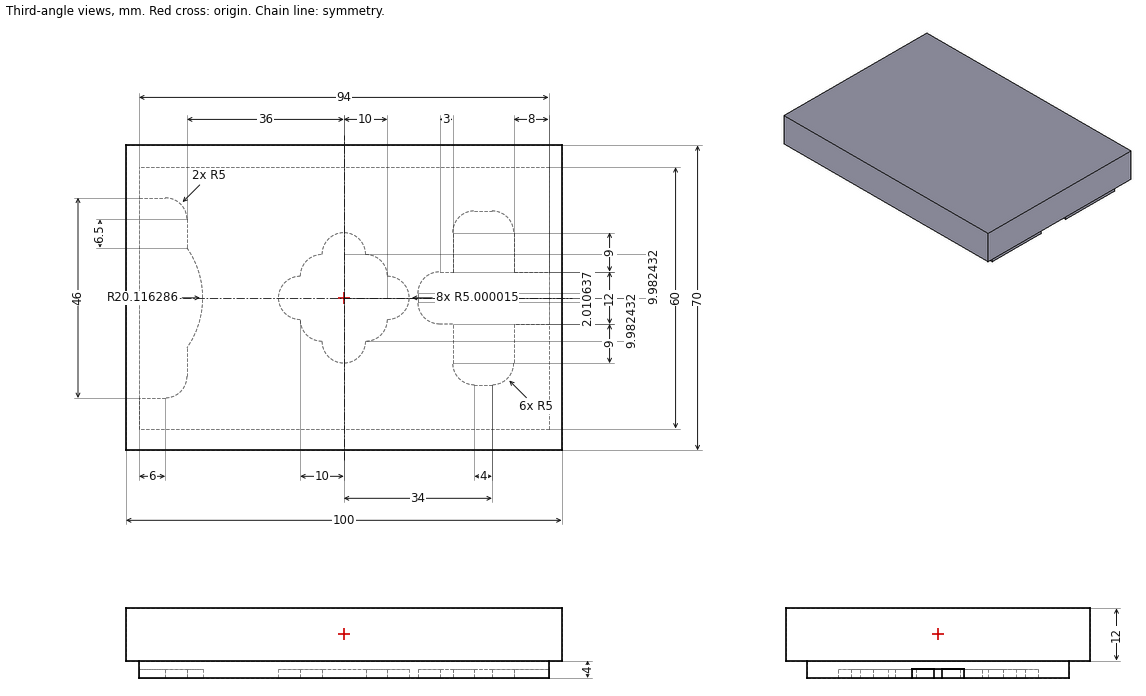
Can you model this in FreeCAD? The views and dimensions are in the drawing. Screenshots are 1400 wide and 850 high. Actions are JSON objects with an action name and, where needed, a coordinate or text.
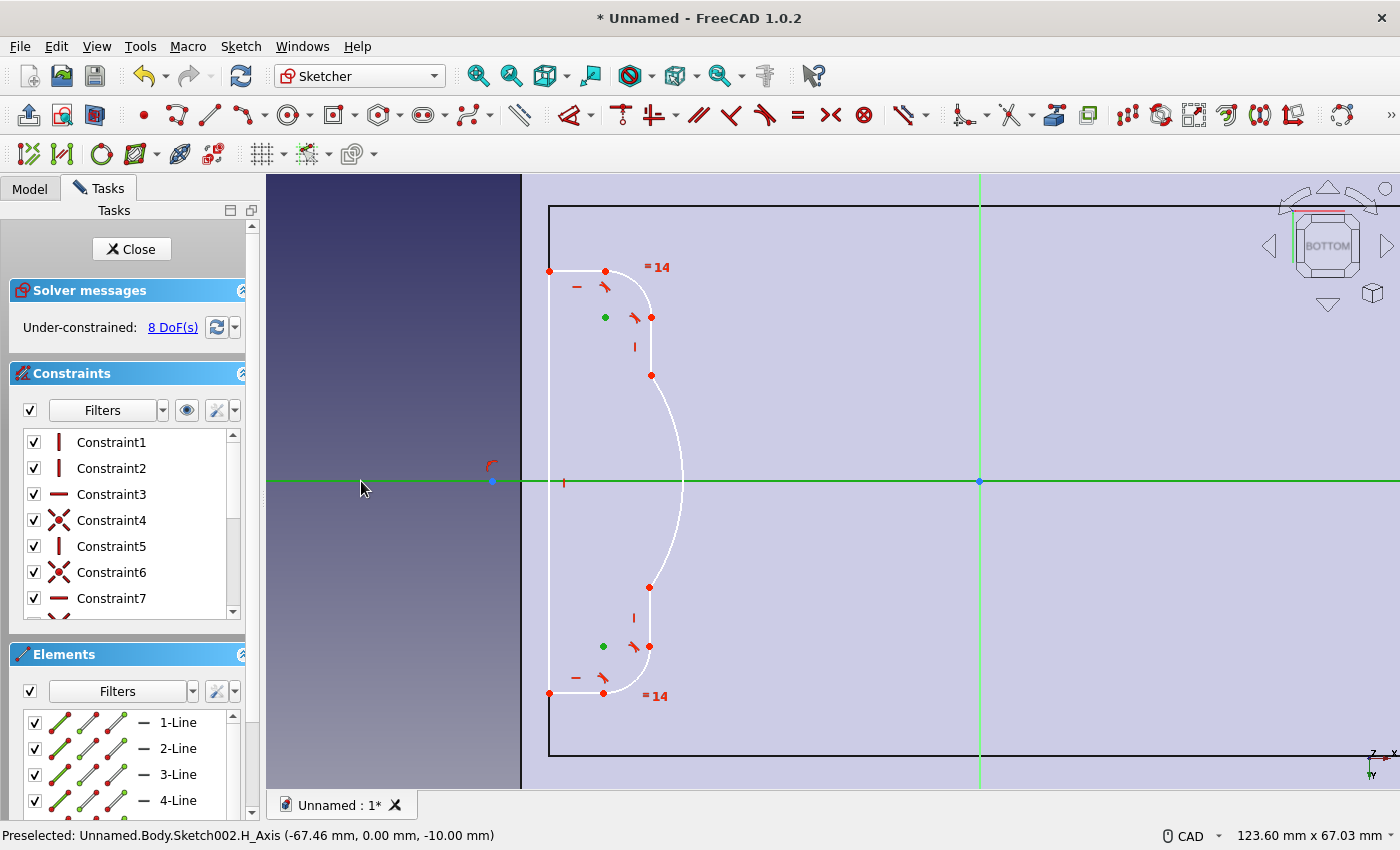
{"action": "left_click", "coordinate": [831, 116]}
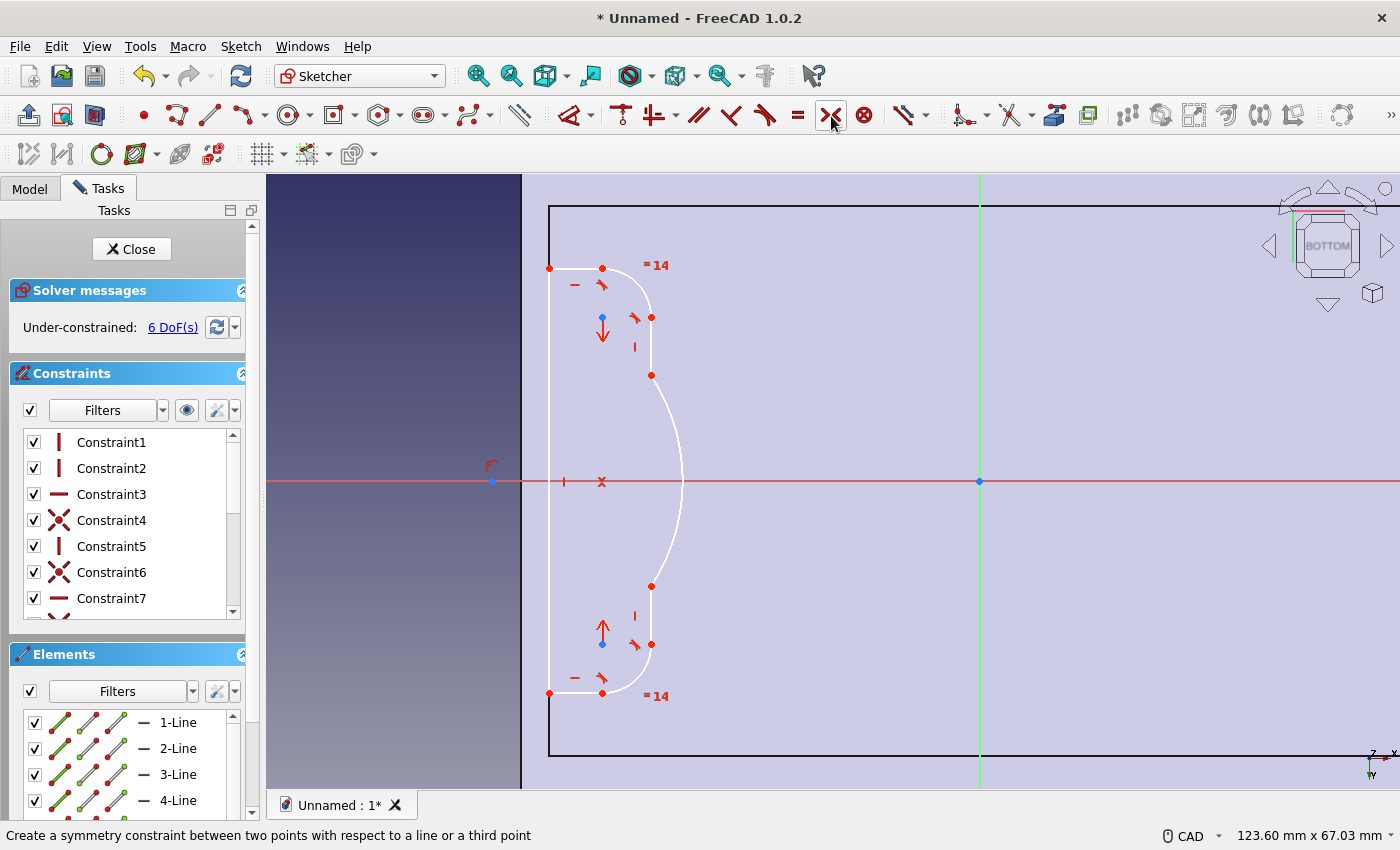
{"action": "left_click", "coordinate": [568, 116]}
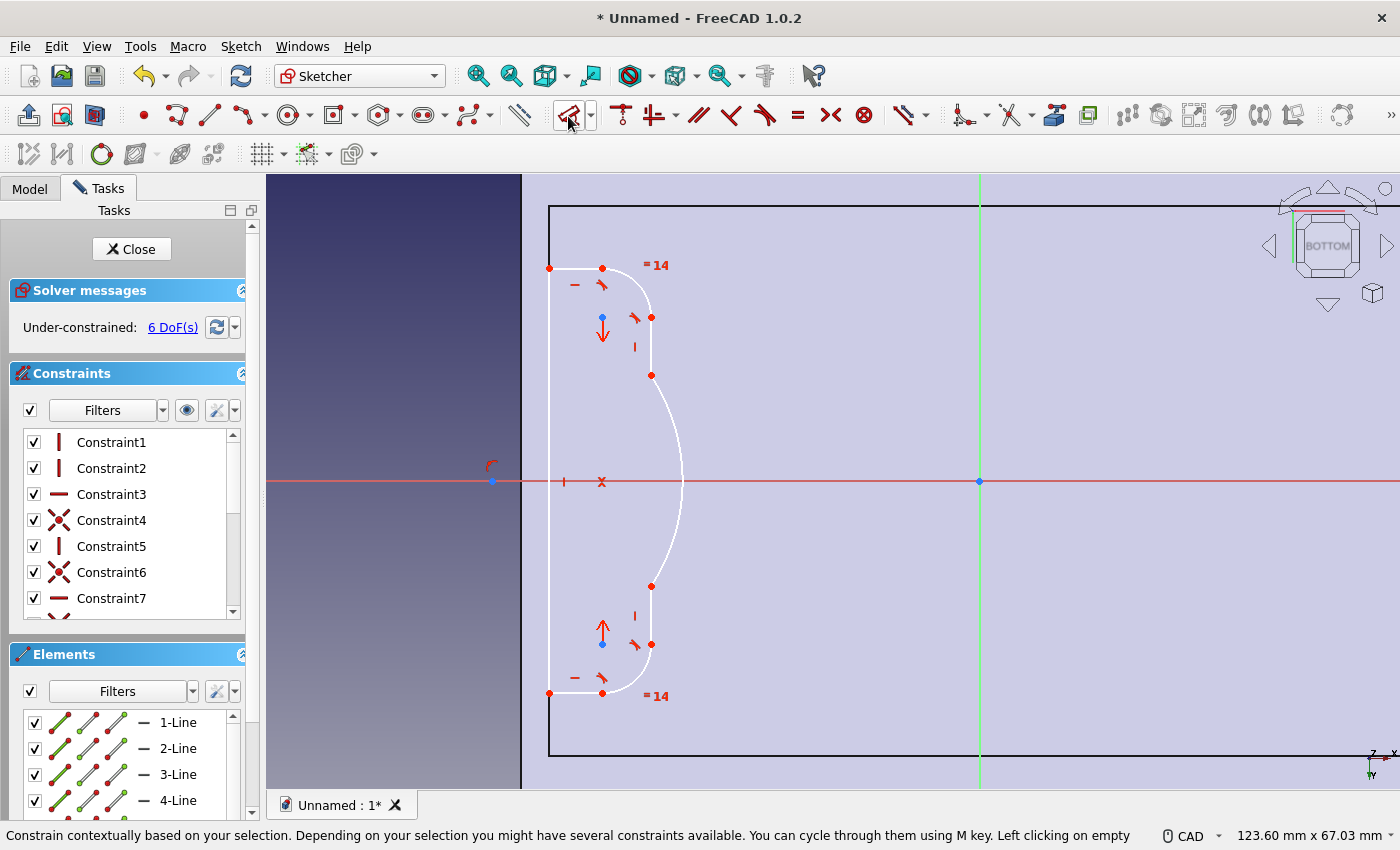
{"action": "left_click", "coordinate": [677, 525]}
{"action": "left_click", "coordinate": [708, 532]}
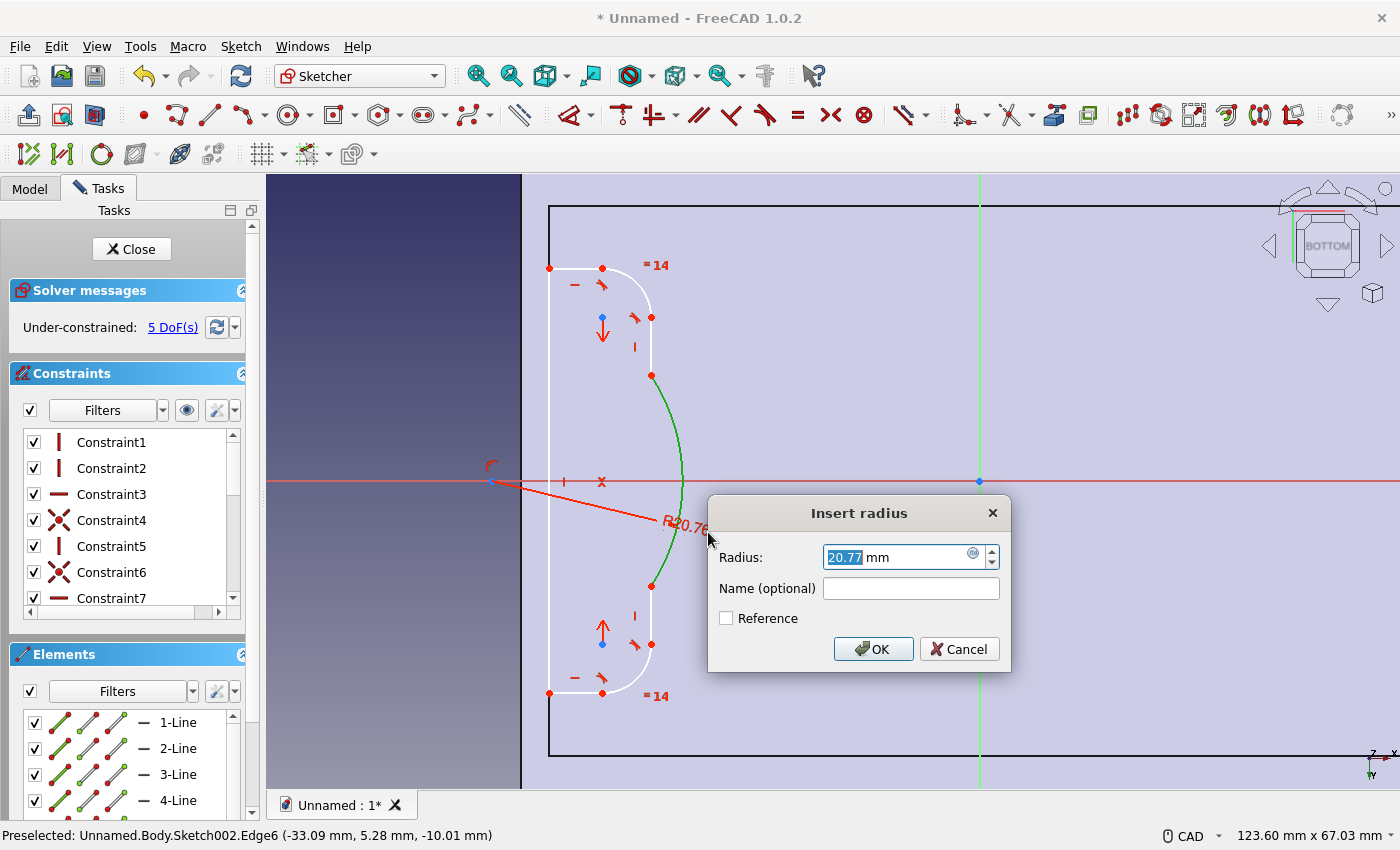
{"action": "type", "text": "20.116286"}
{"action": "key", "text": "Return"}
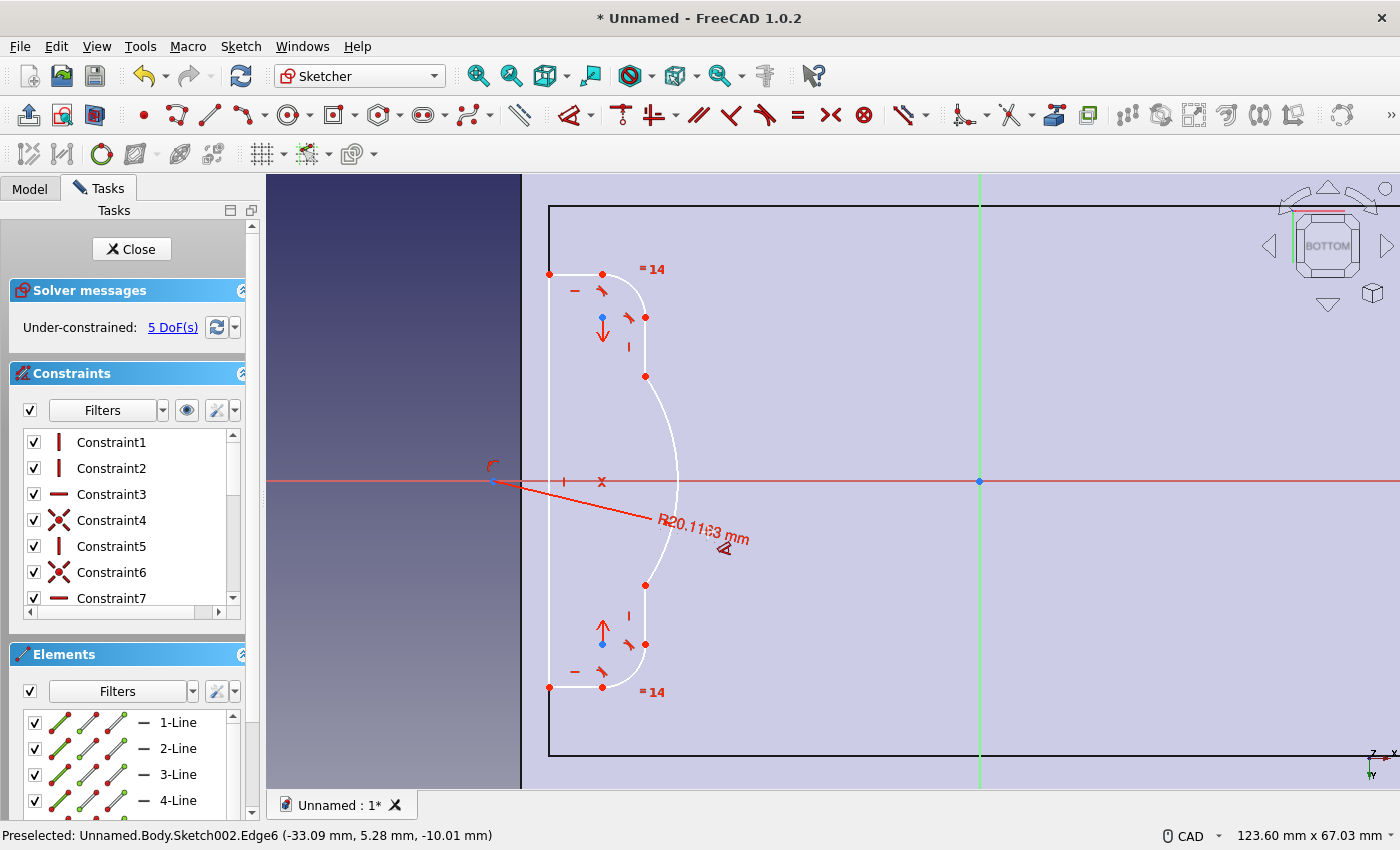
{"action": "left_click", "coordinate": [641, 298]}
{"action": "left_click", "coordinate": [670, 284]}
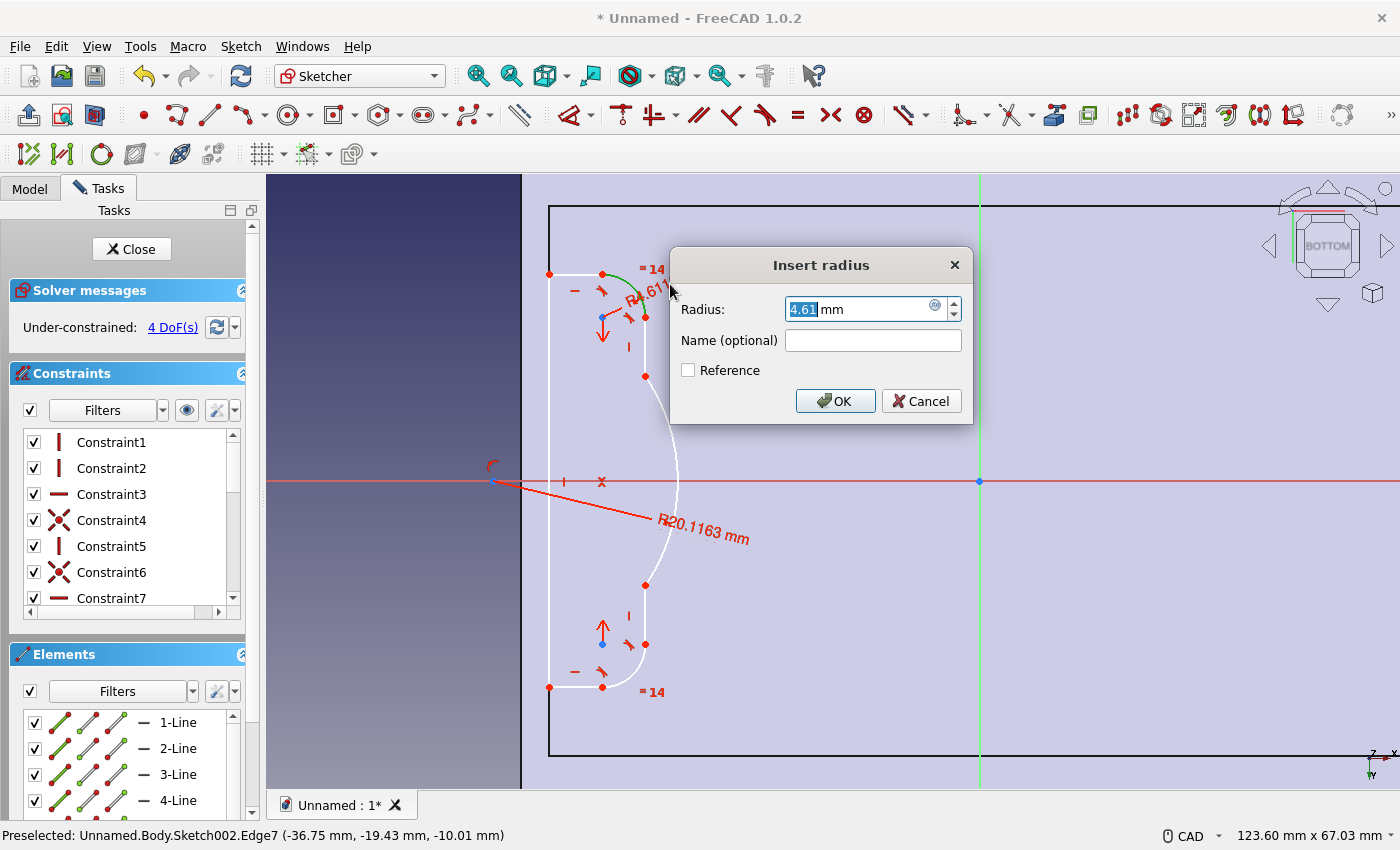
{"action": "type", "text": "5"}
{"action": "key", "text": "Return"}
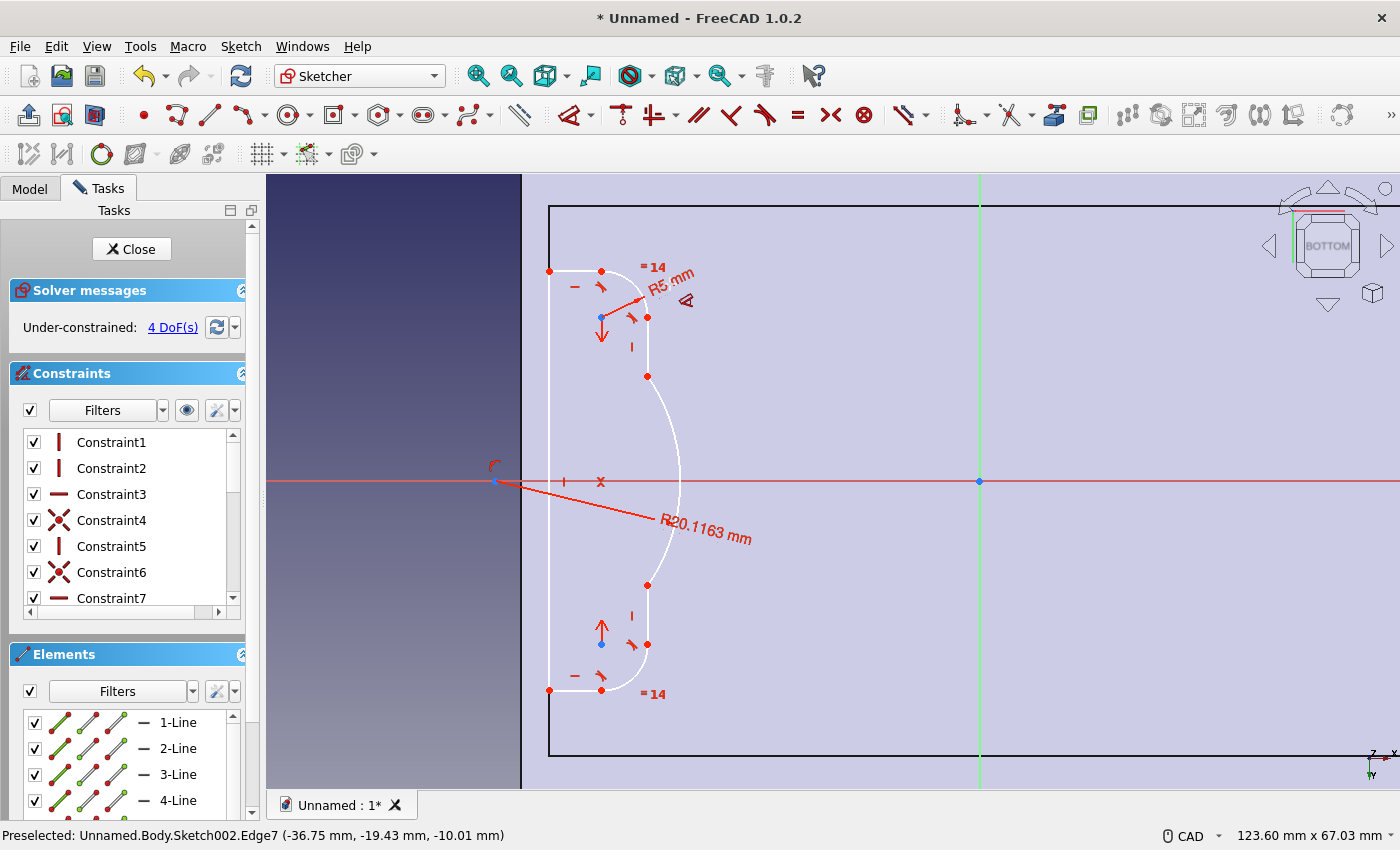
{"action": "left_click", "coordinate": [586, 271]}
{"action": "left_click", "coordinate": [575, 237]}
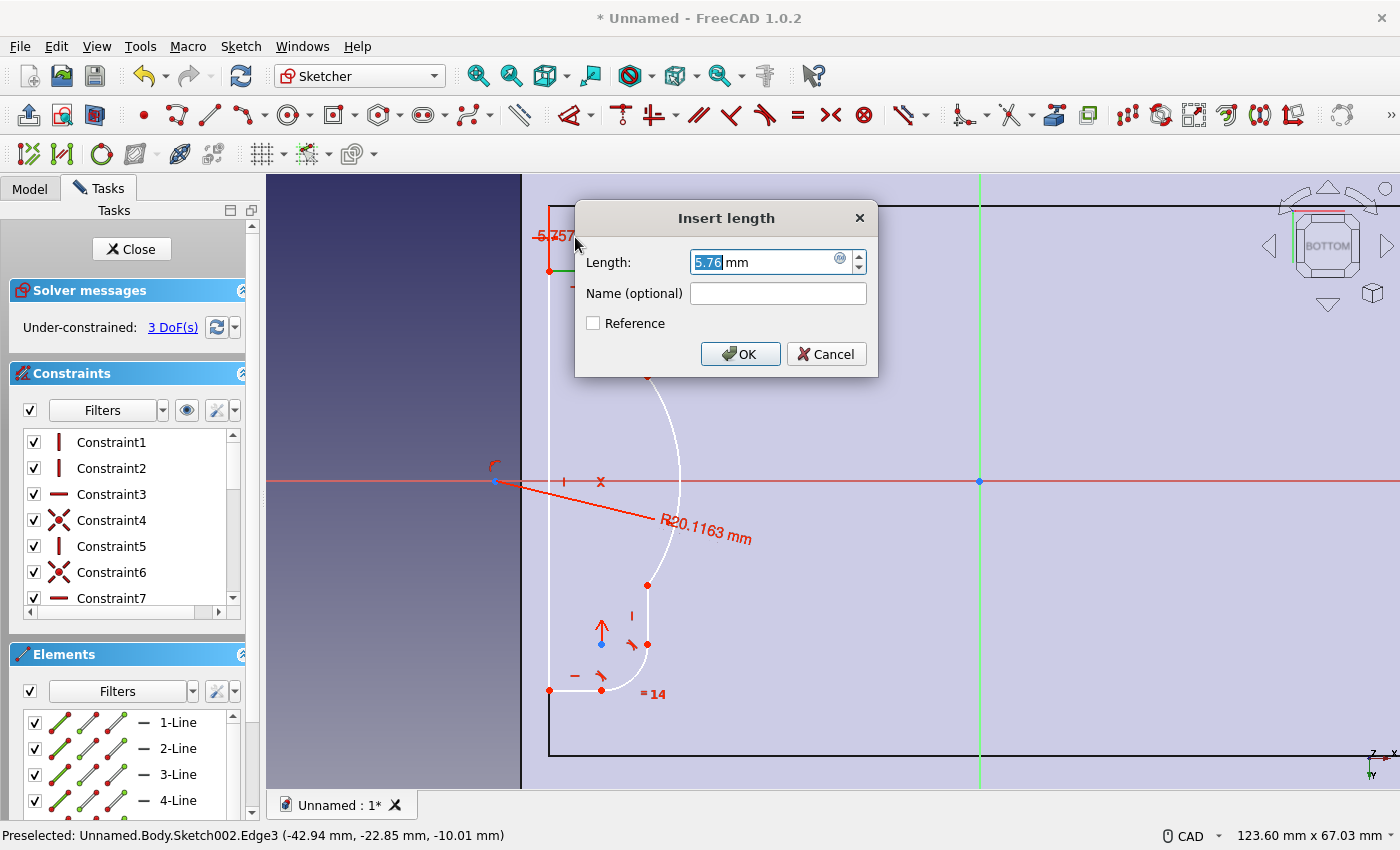
{"action": "type", "text": "6"}
{"action": "key", "text": "Return"}